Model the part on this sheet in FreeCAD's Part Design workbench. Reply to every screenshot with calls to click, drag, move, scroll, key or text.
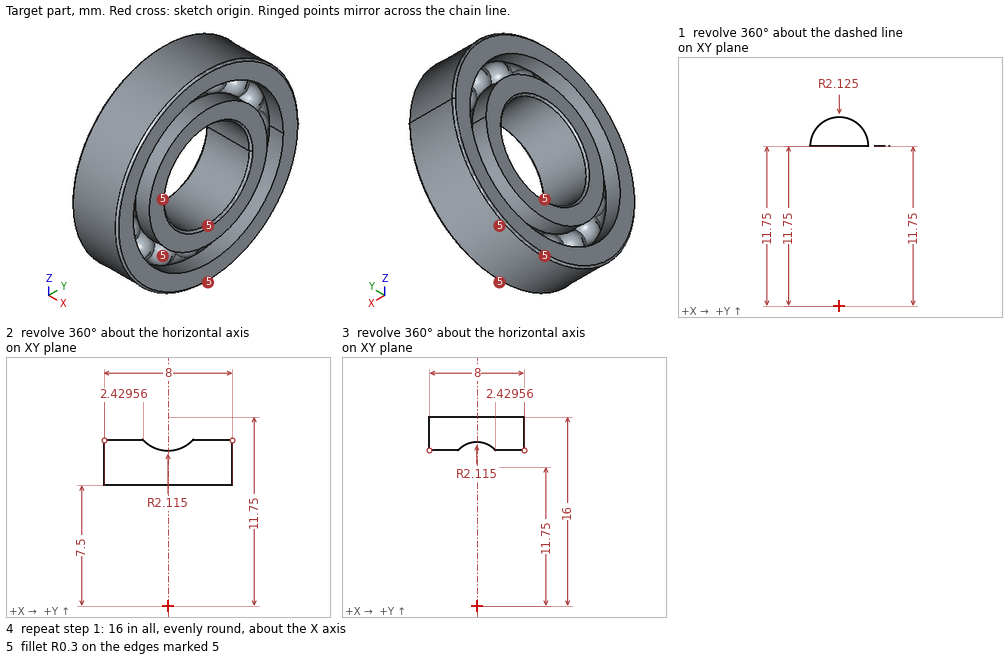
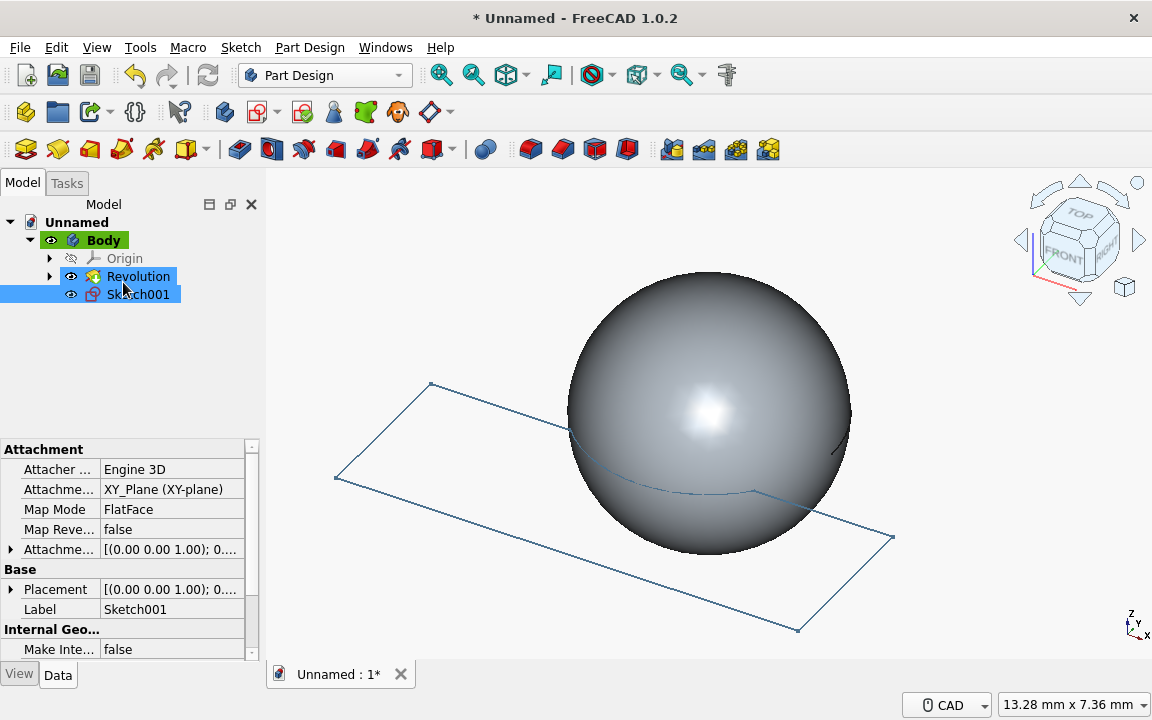
click(58, 150)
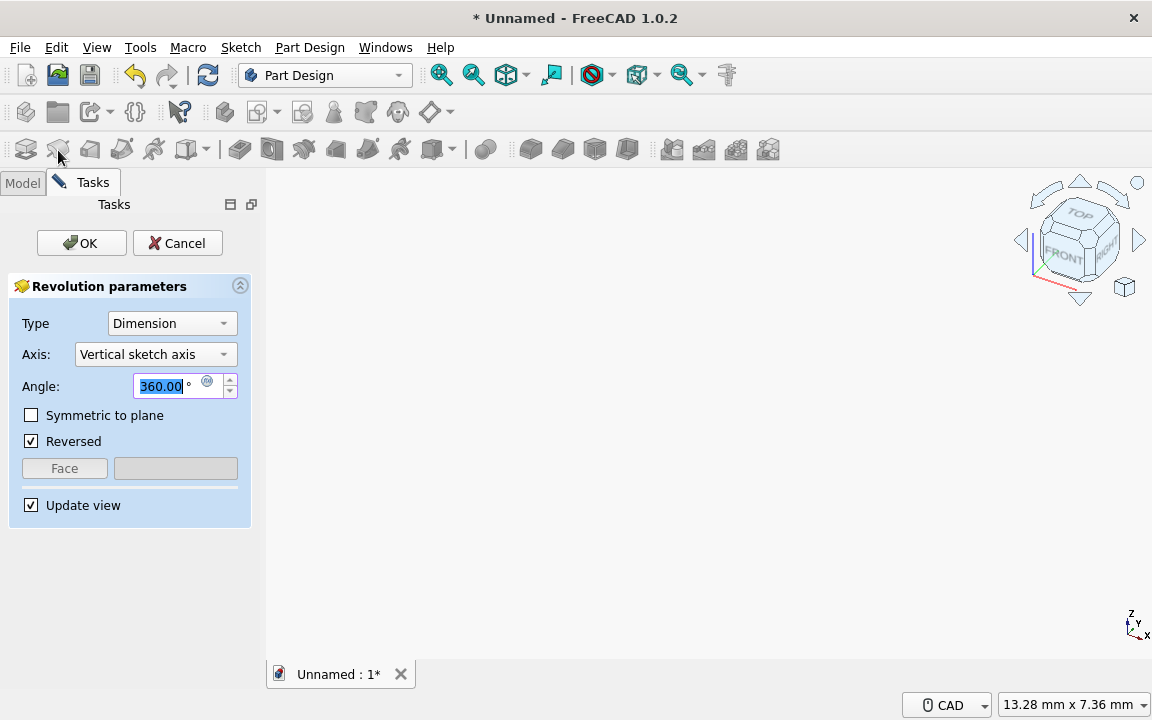
click(156, 354)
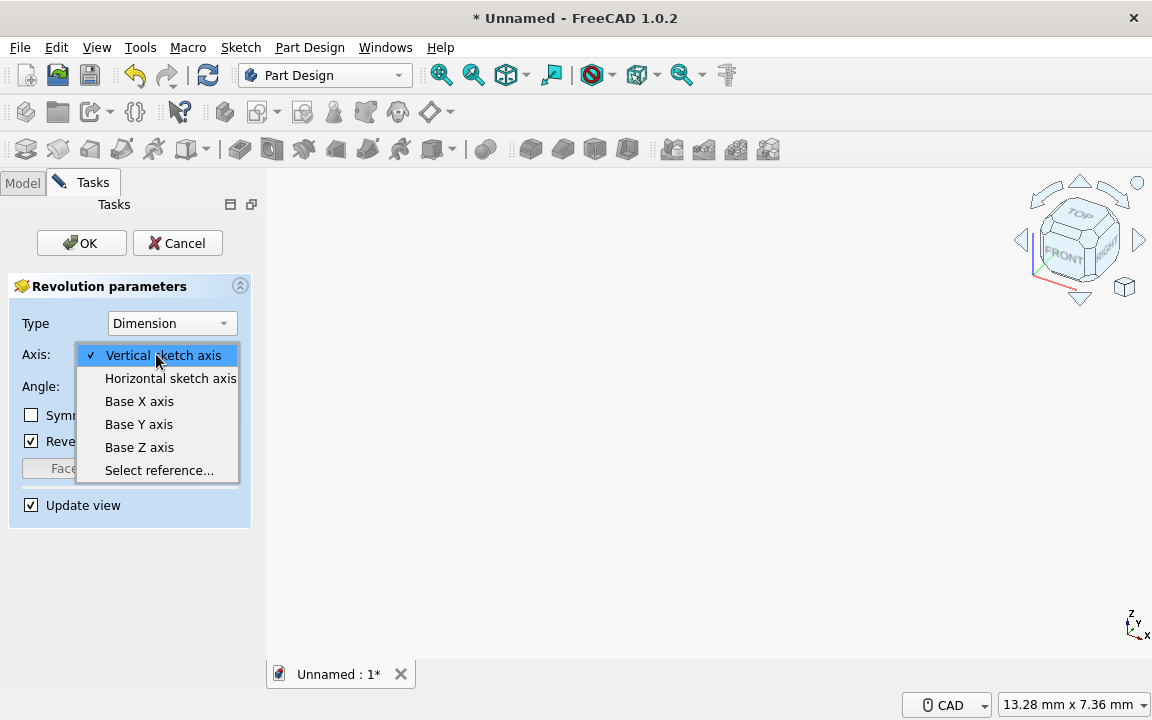
click(156, 378)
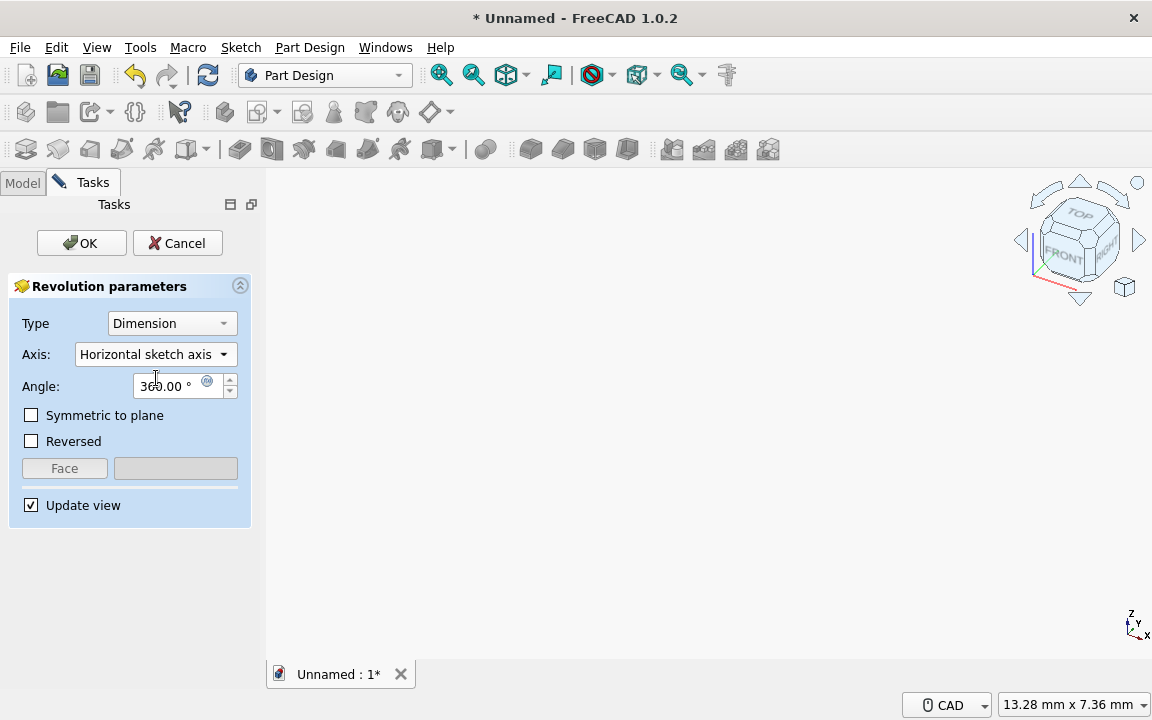
click(82, 243)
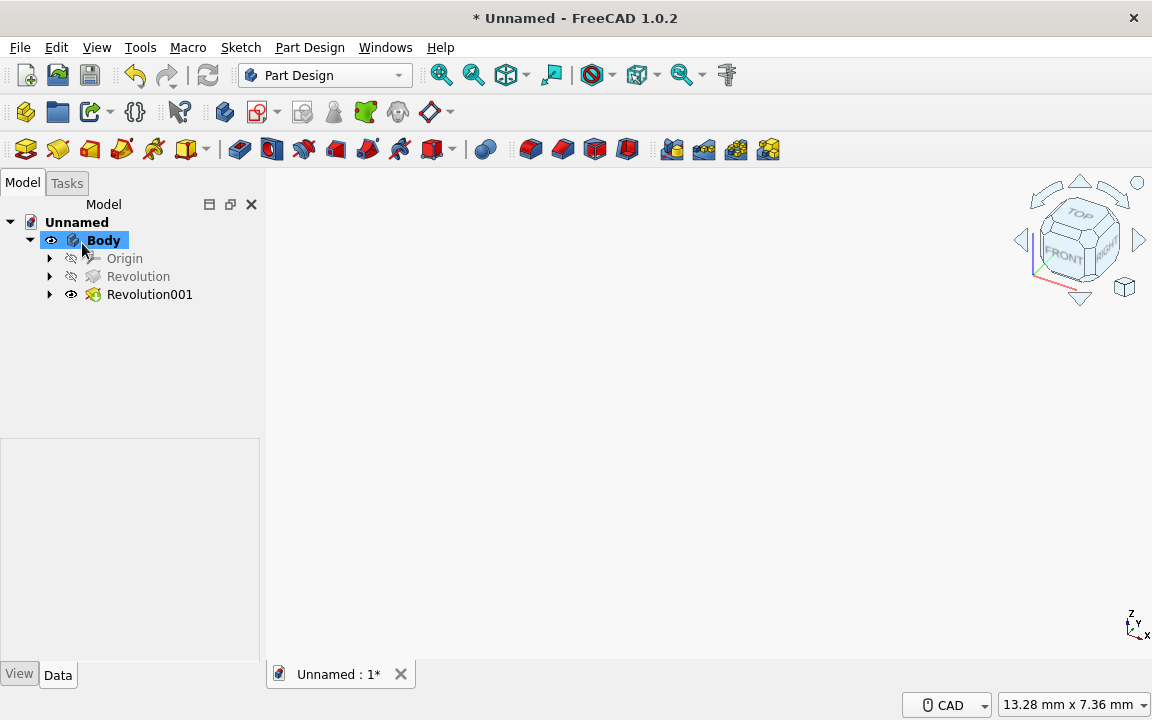
click(442, 76)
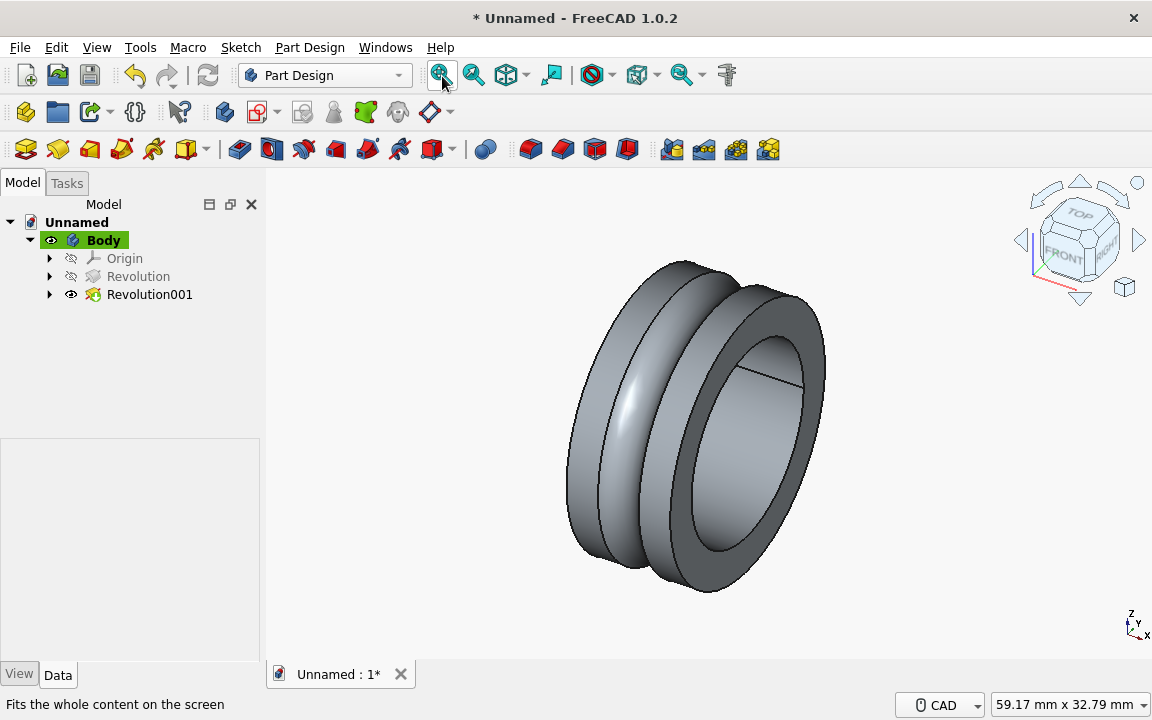
click(258, 112)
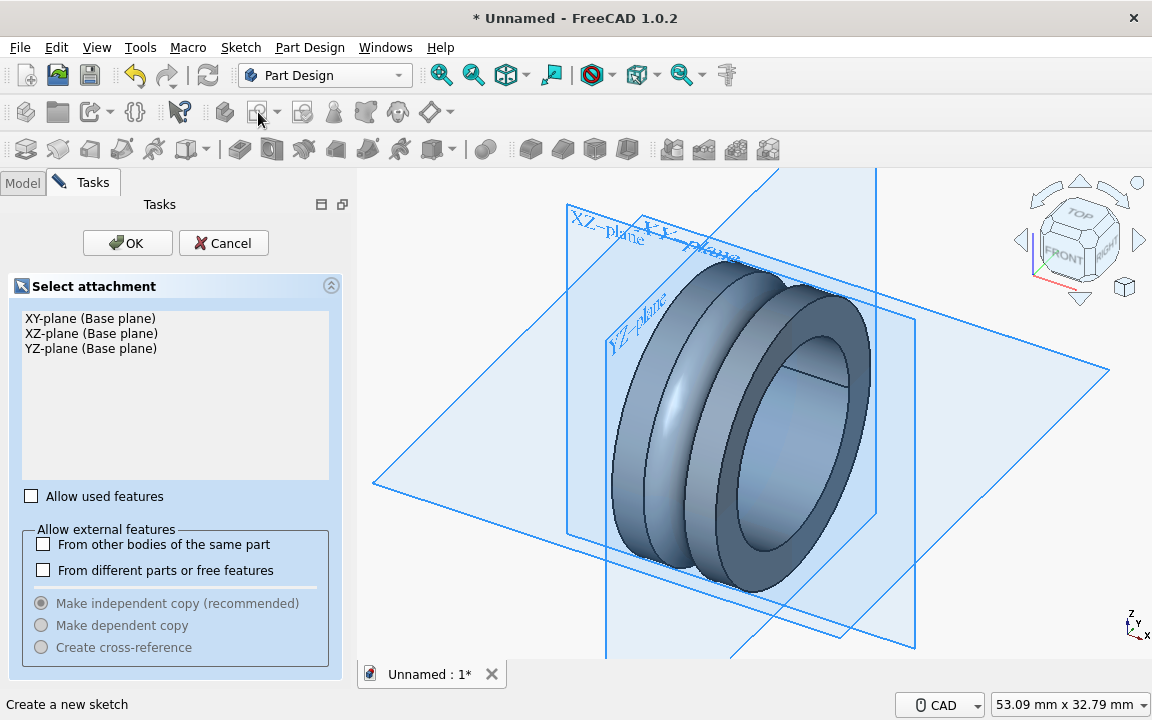
click(82, 318)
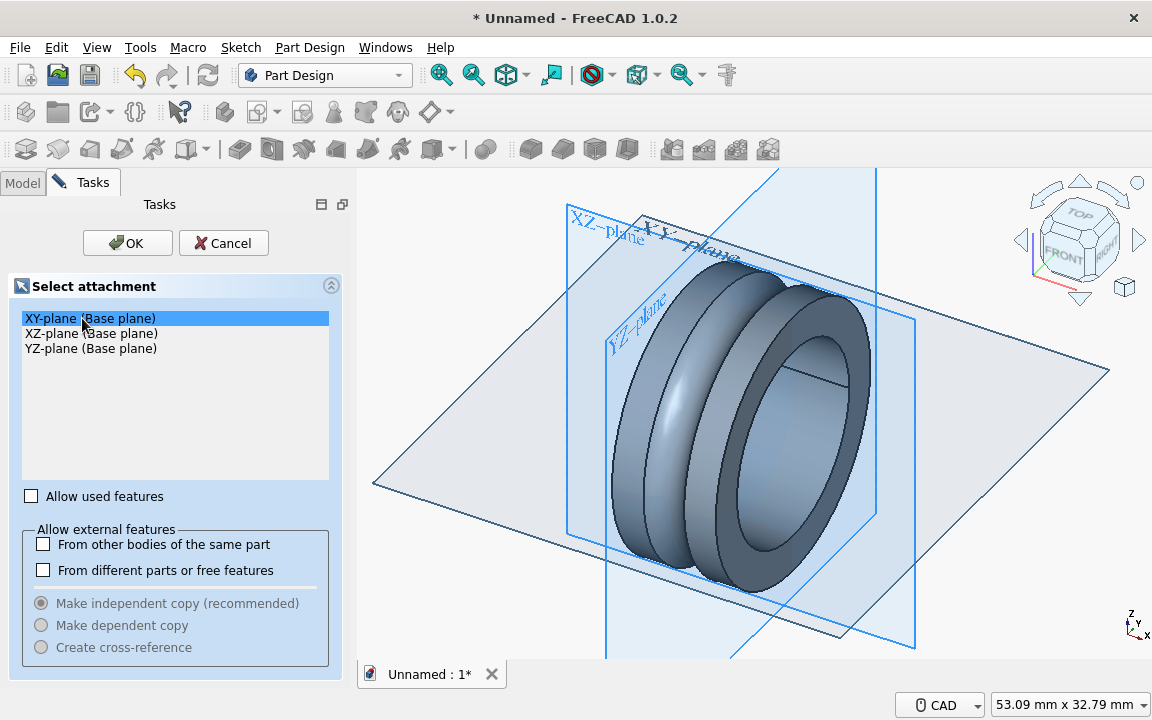
click(128, 243)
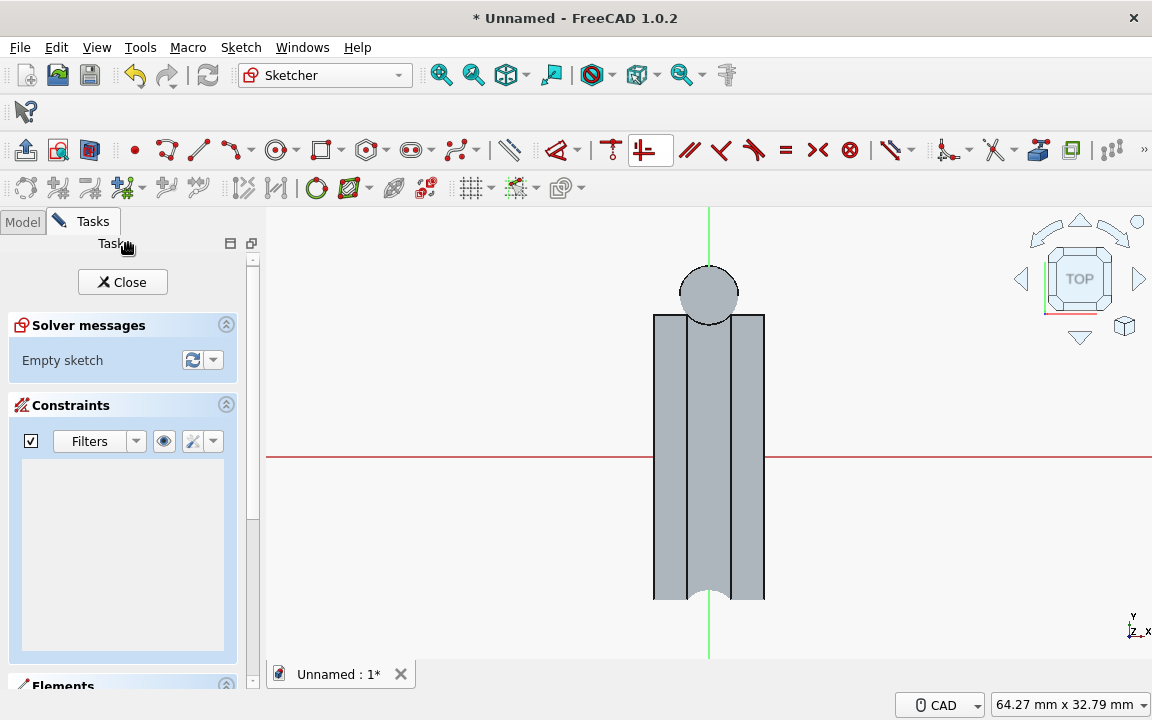
click(90, 150)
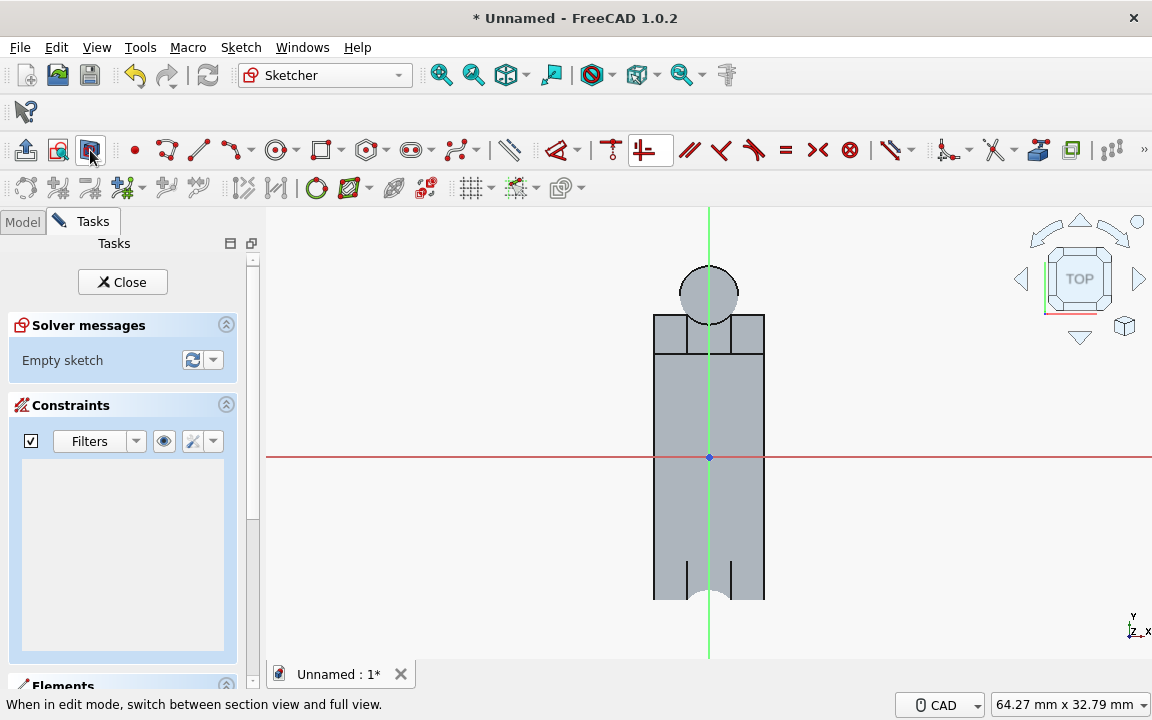
scroll(331, 631, down, 1)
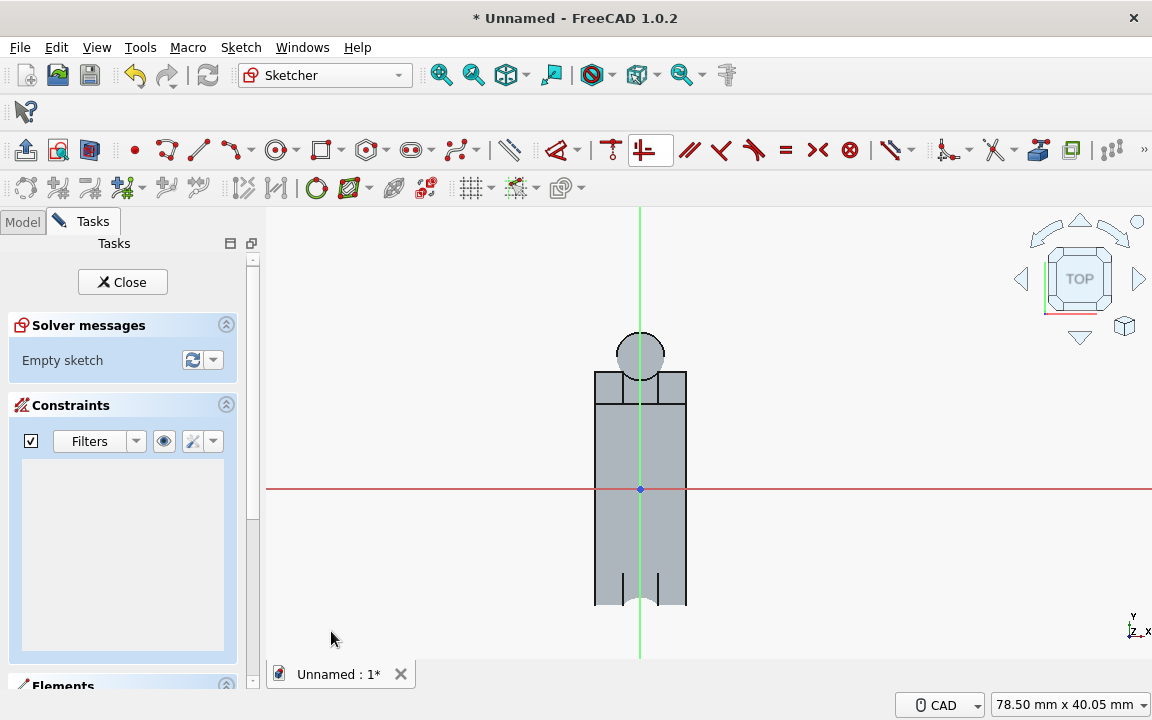
scroll(640, 329, up, 2)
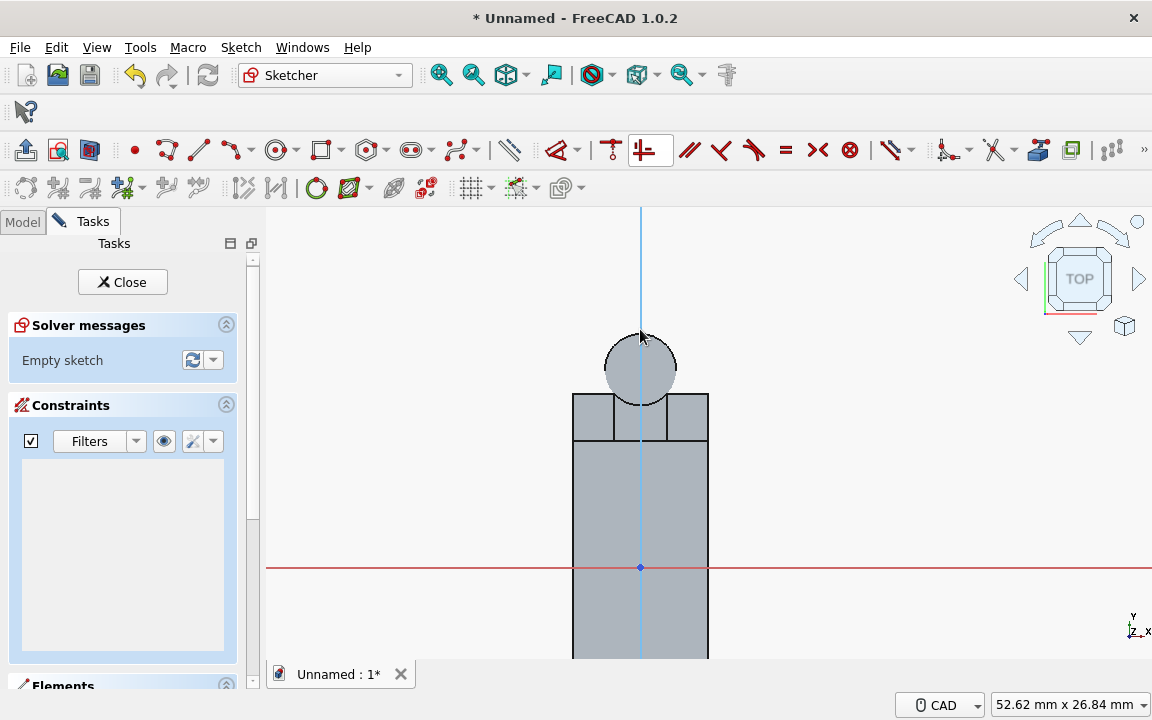
click(168, 150)